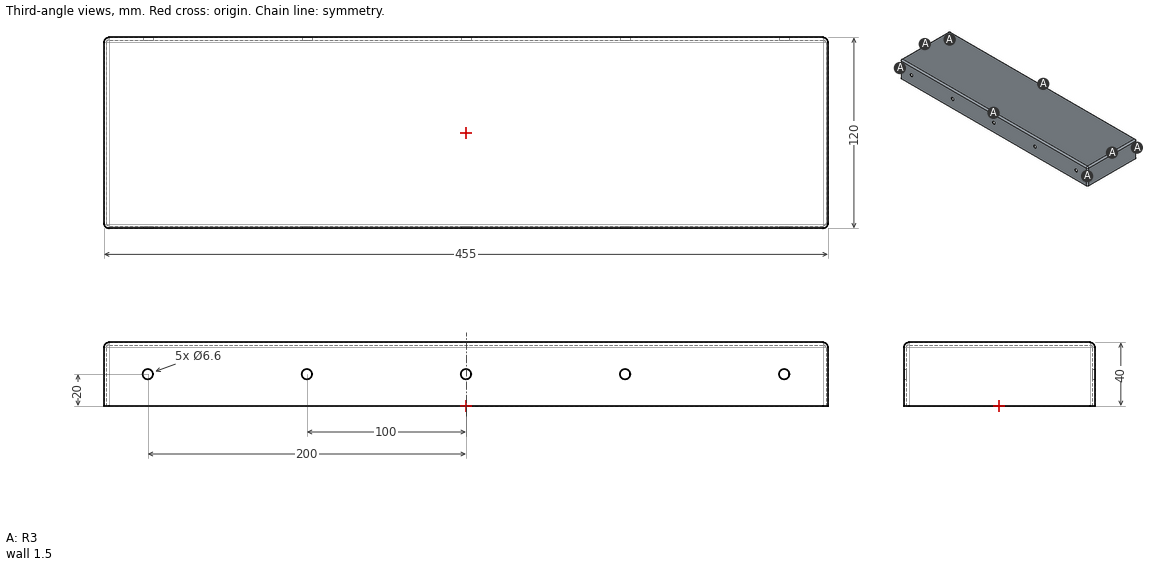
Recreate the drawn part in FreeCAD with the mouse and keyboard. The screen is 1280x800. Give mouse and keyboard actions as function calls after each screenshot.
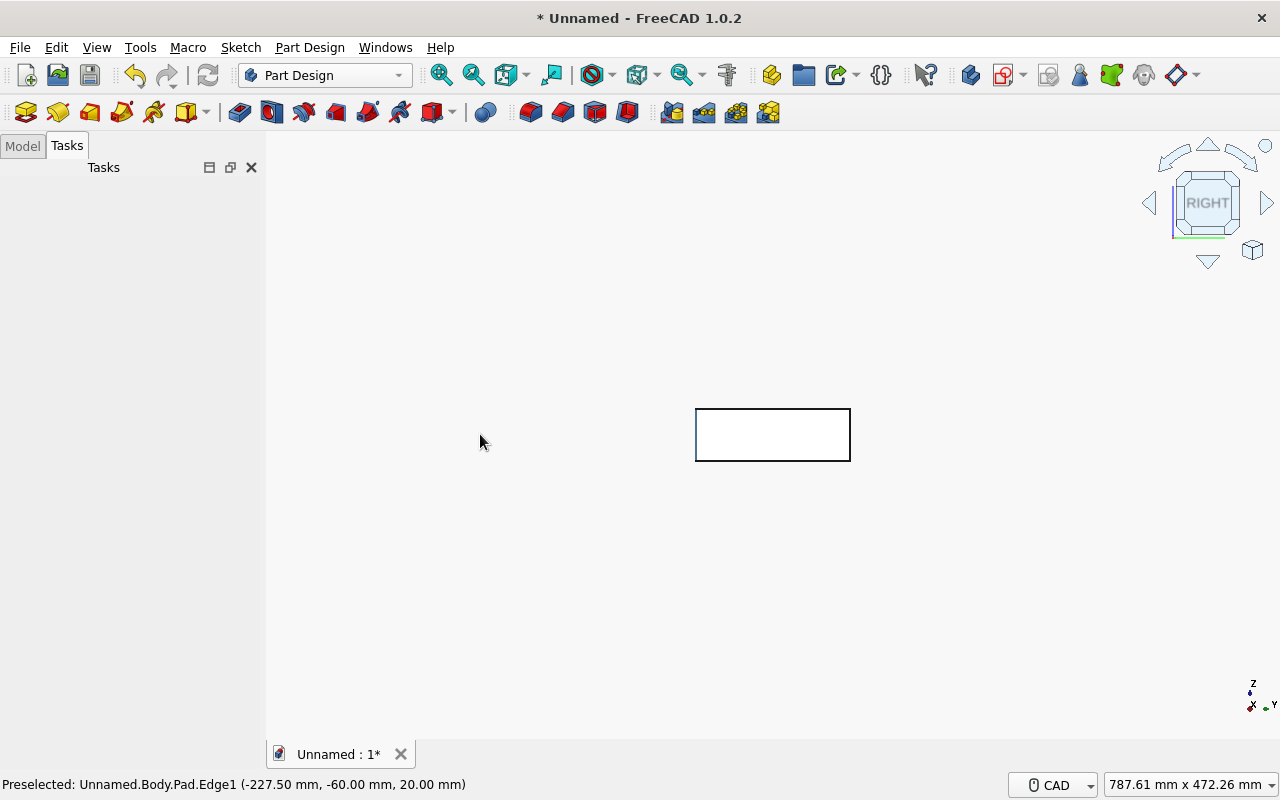
key(v)
key(f)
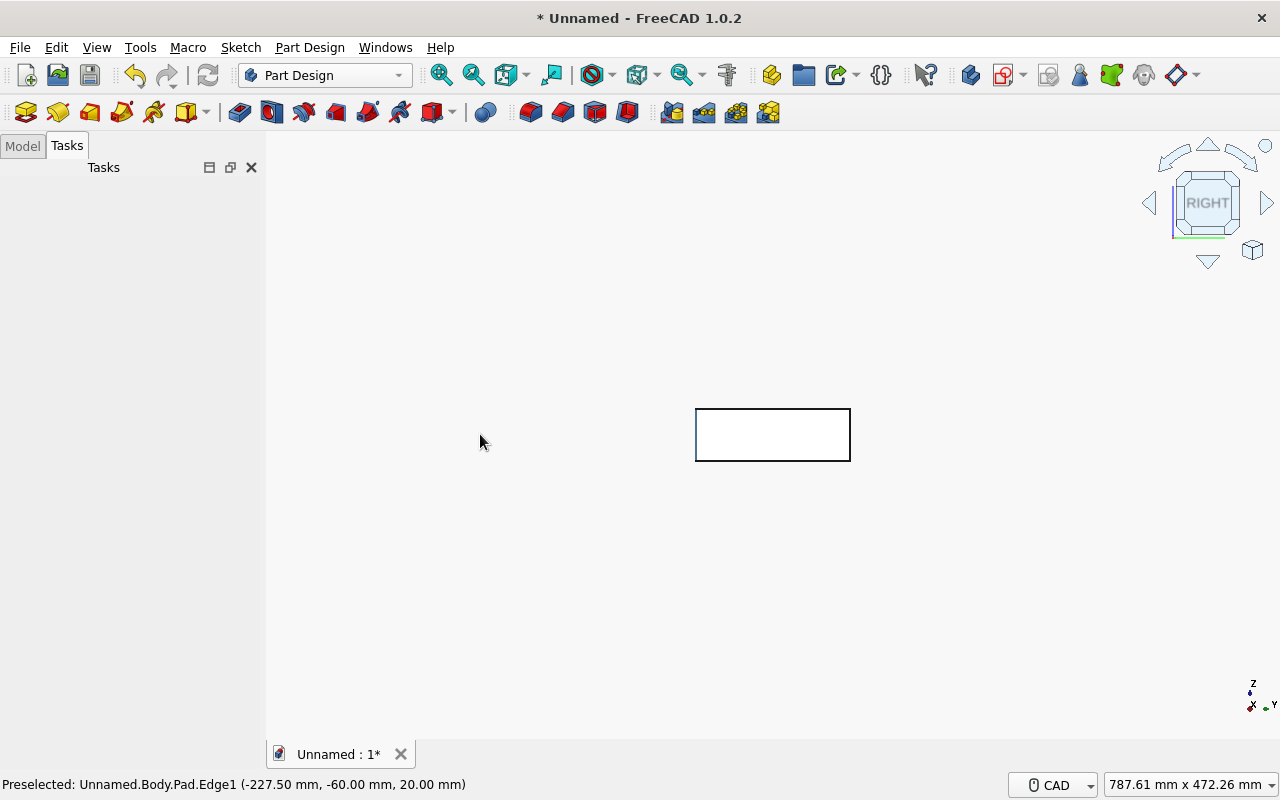
click(850, 434, ctrl)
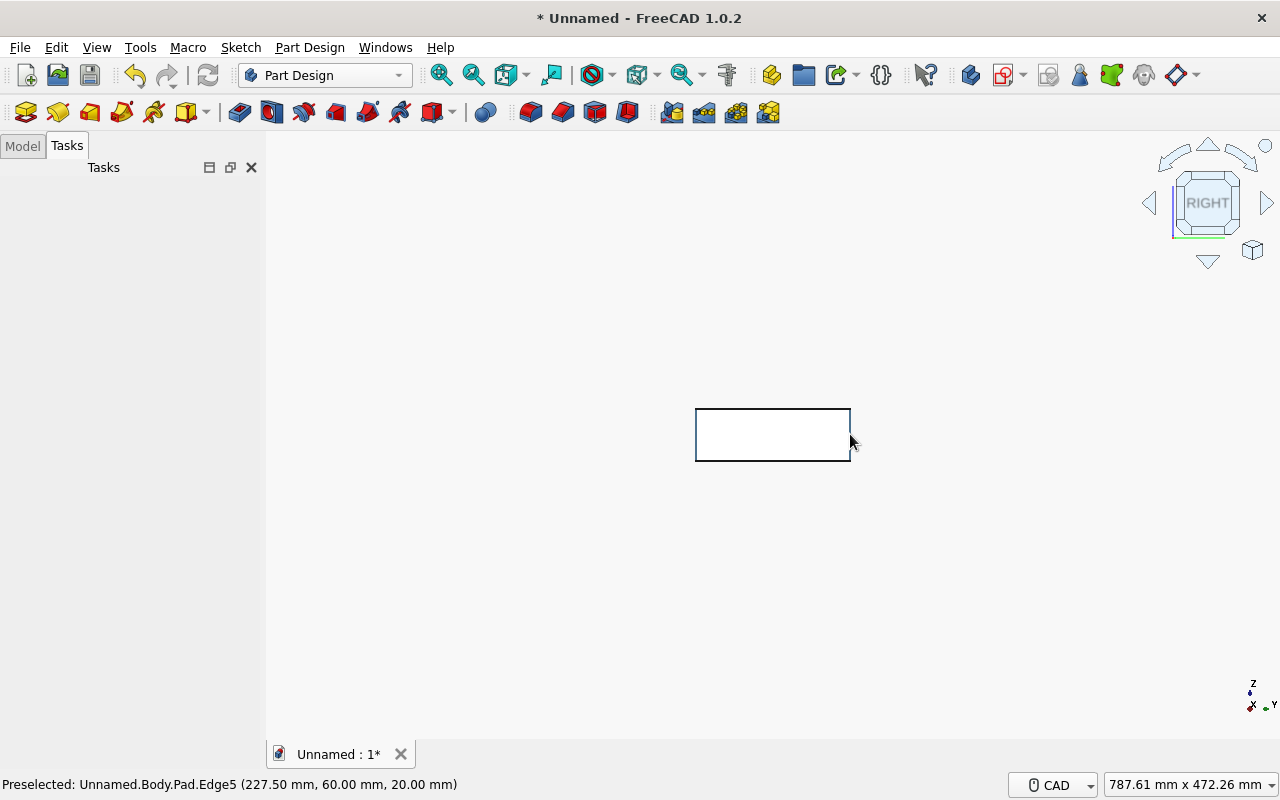
key(5)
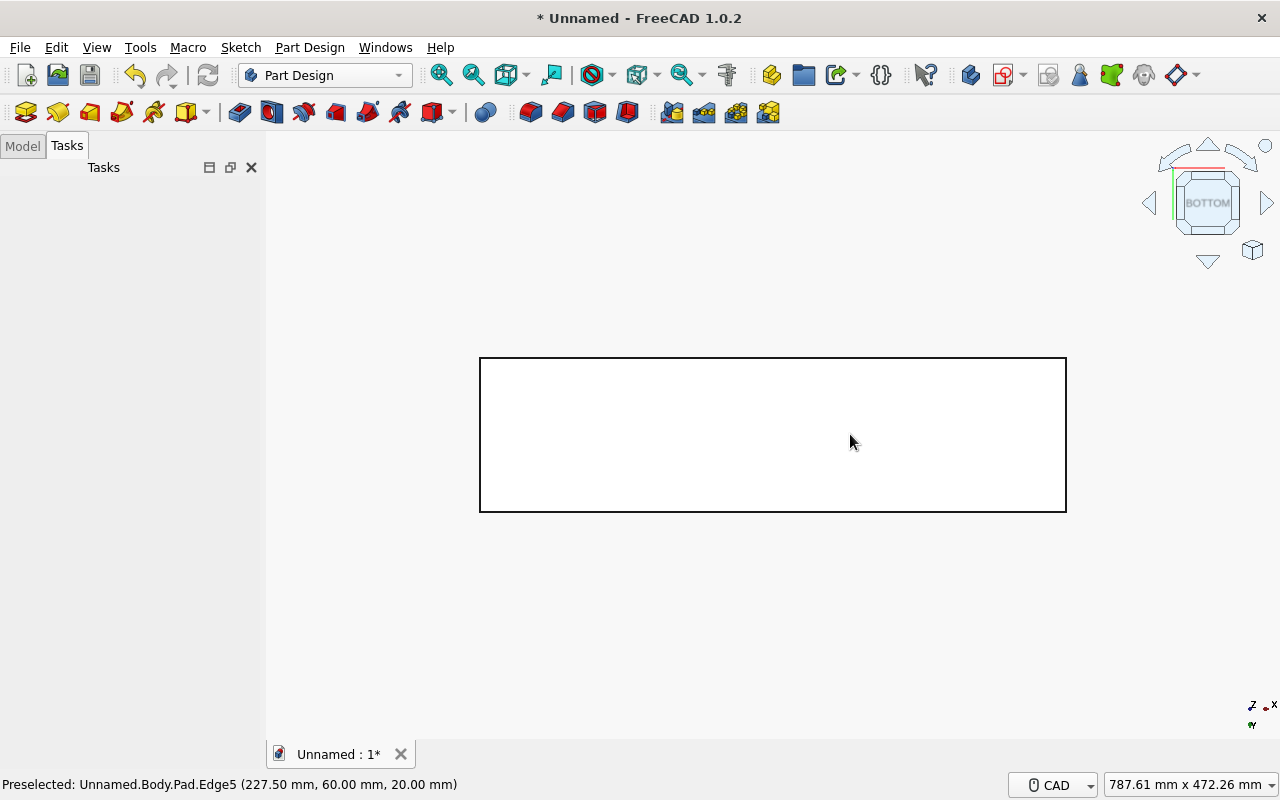
key(4)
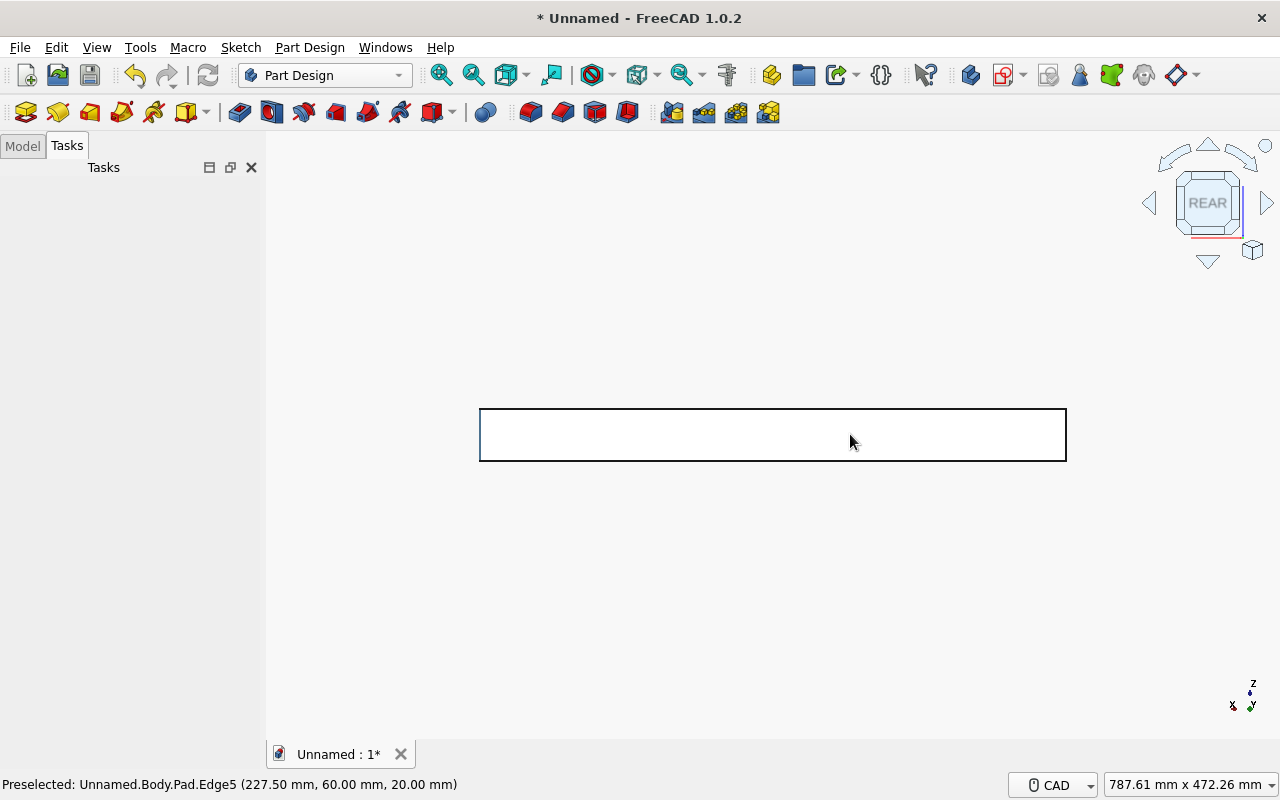
click(1066, 434, ctrl)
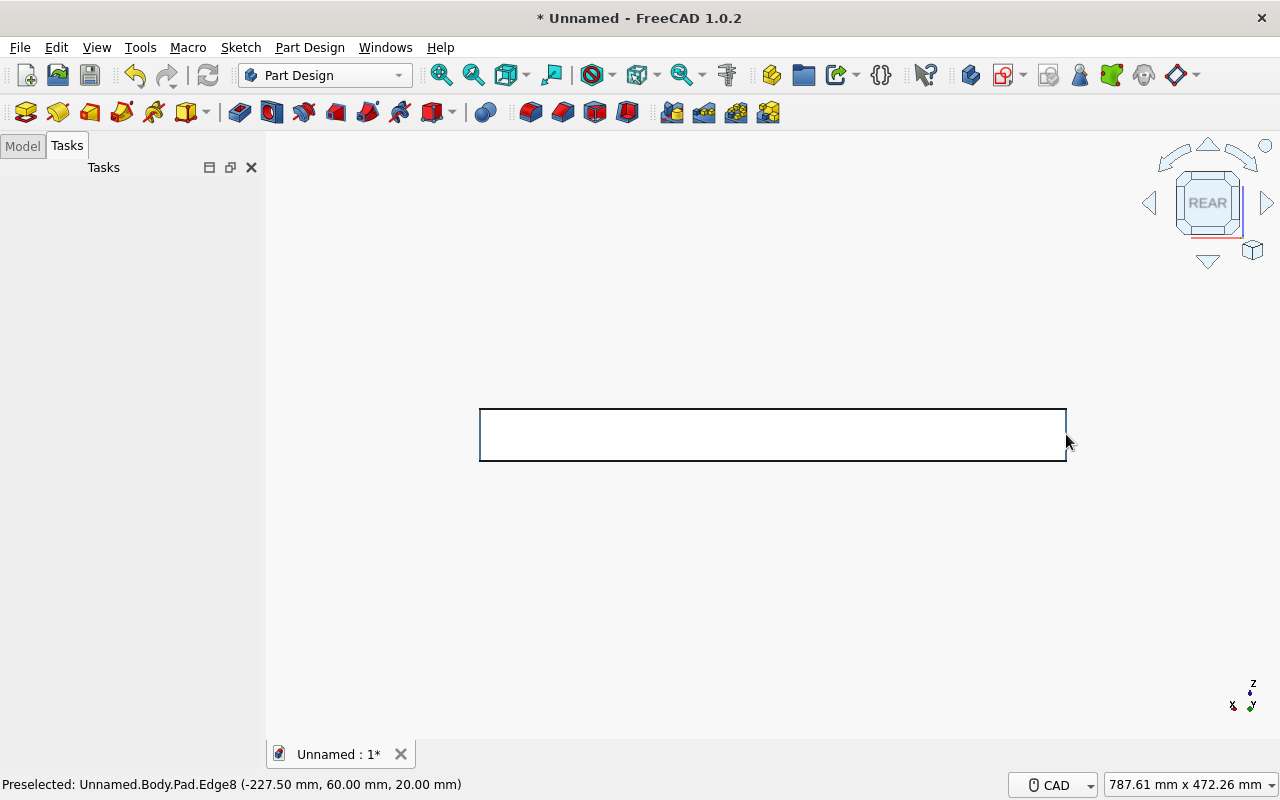
click(532, 112)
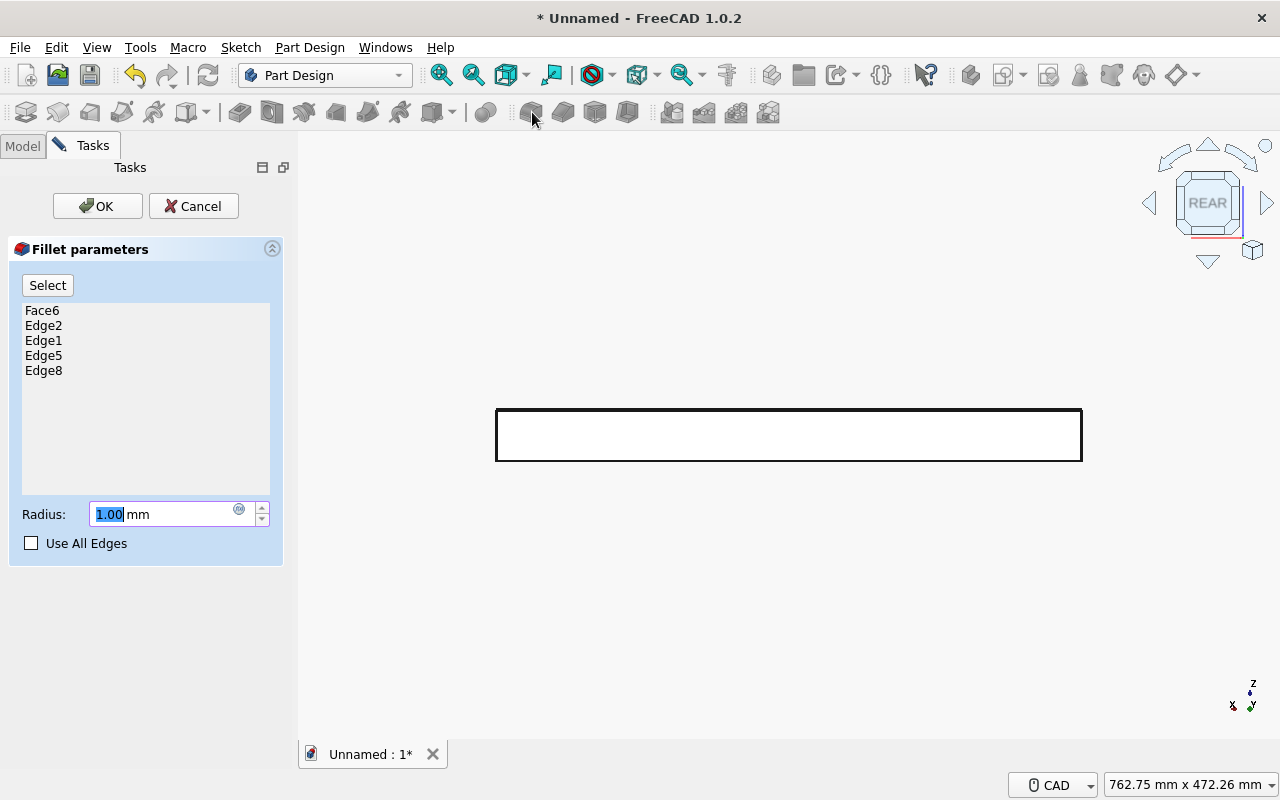
text(3)
key(Tab)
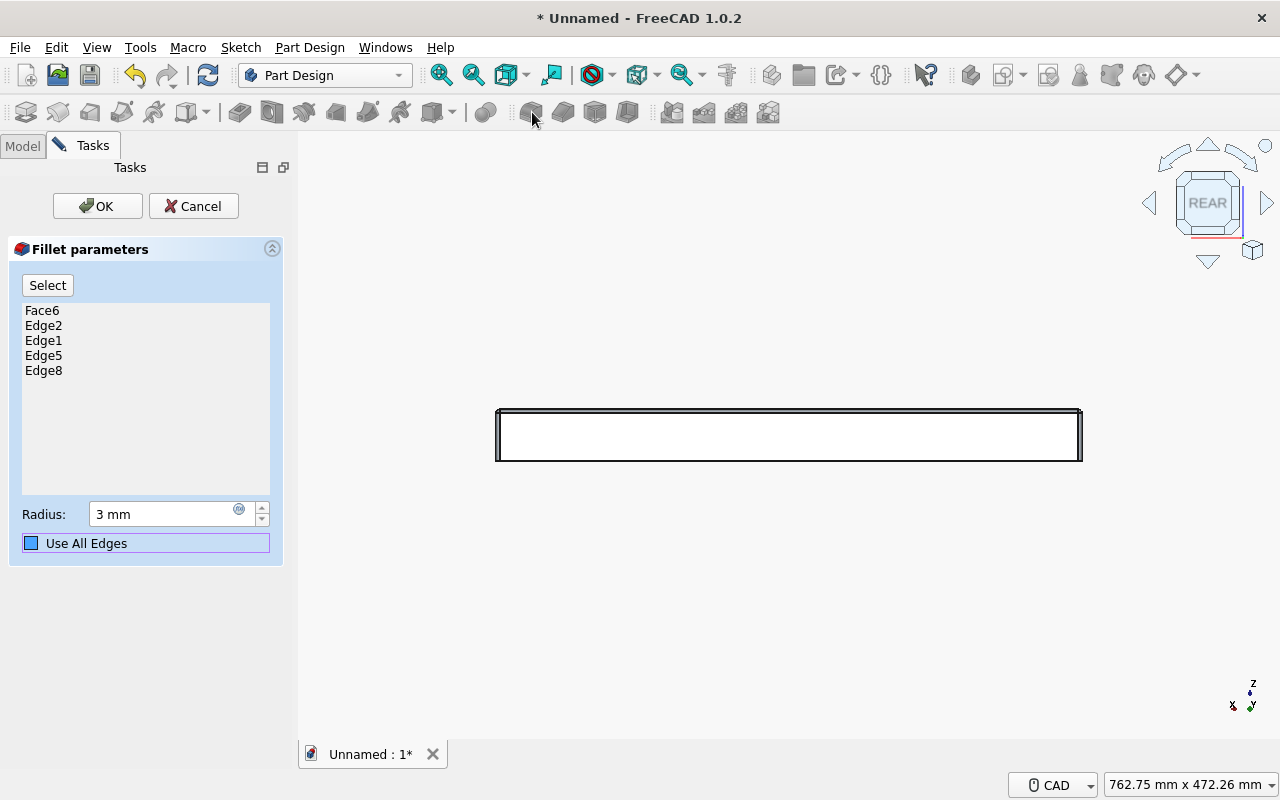
click(98, 206)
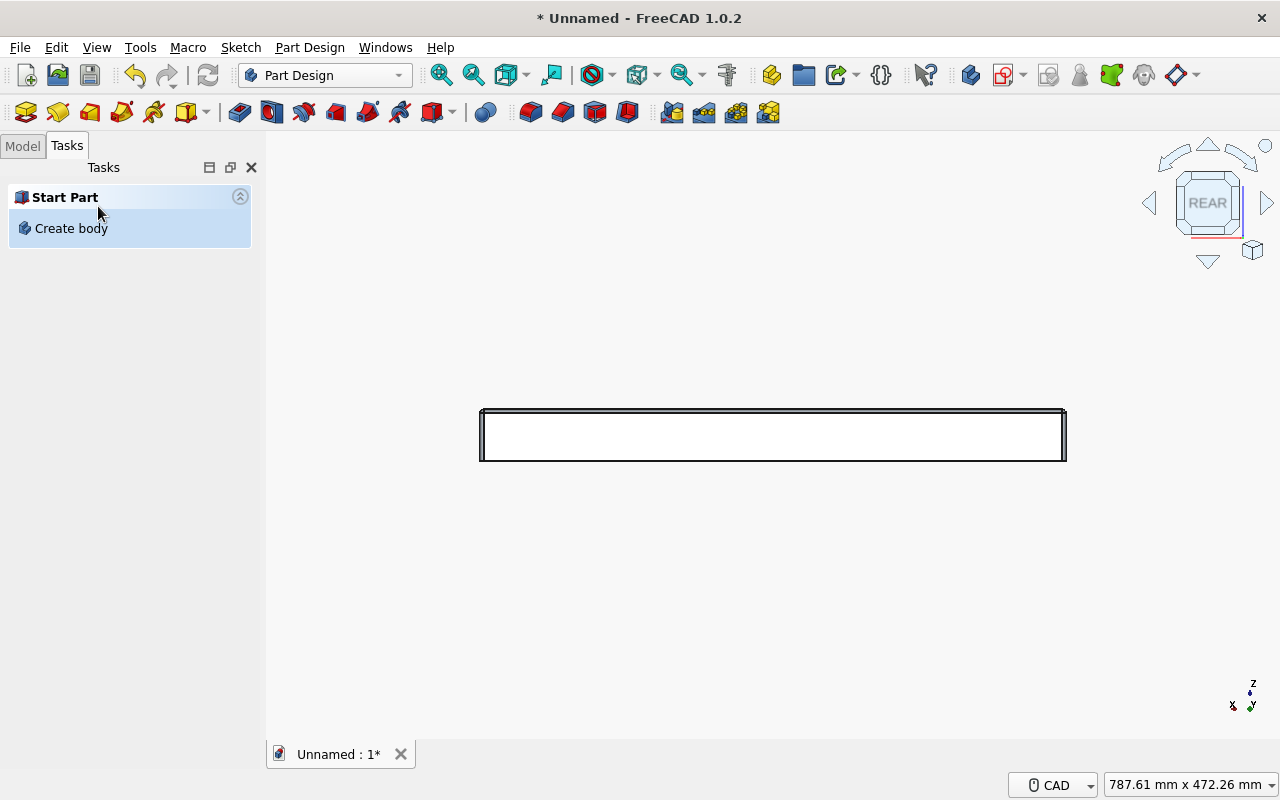
key(0)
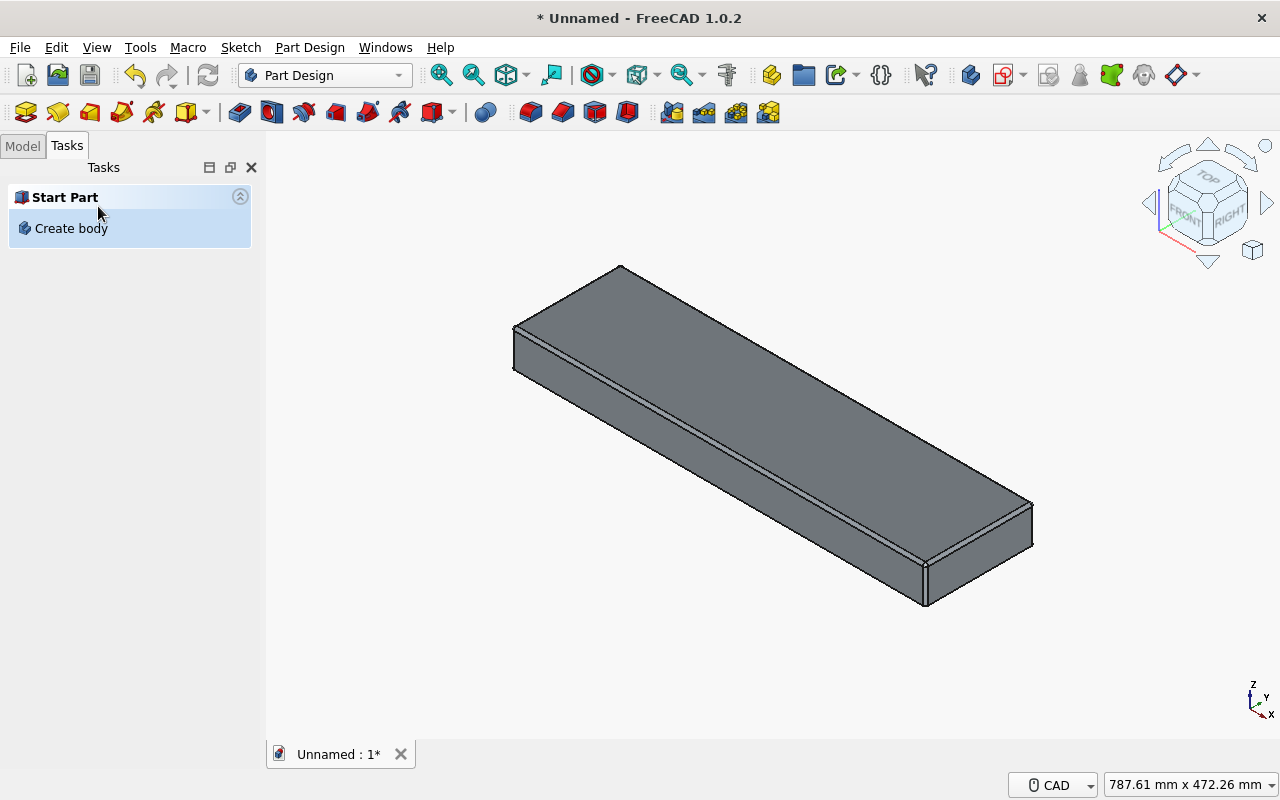
key(2)